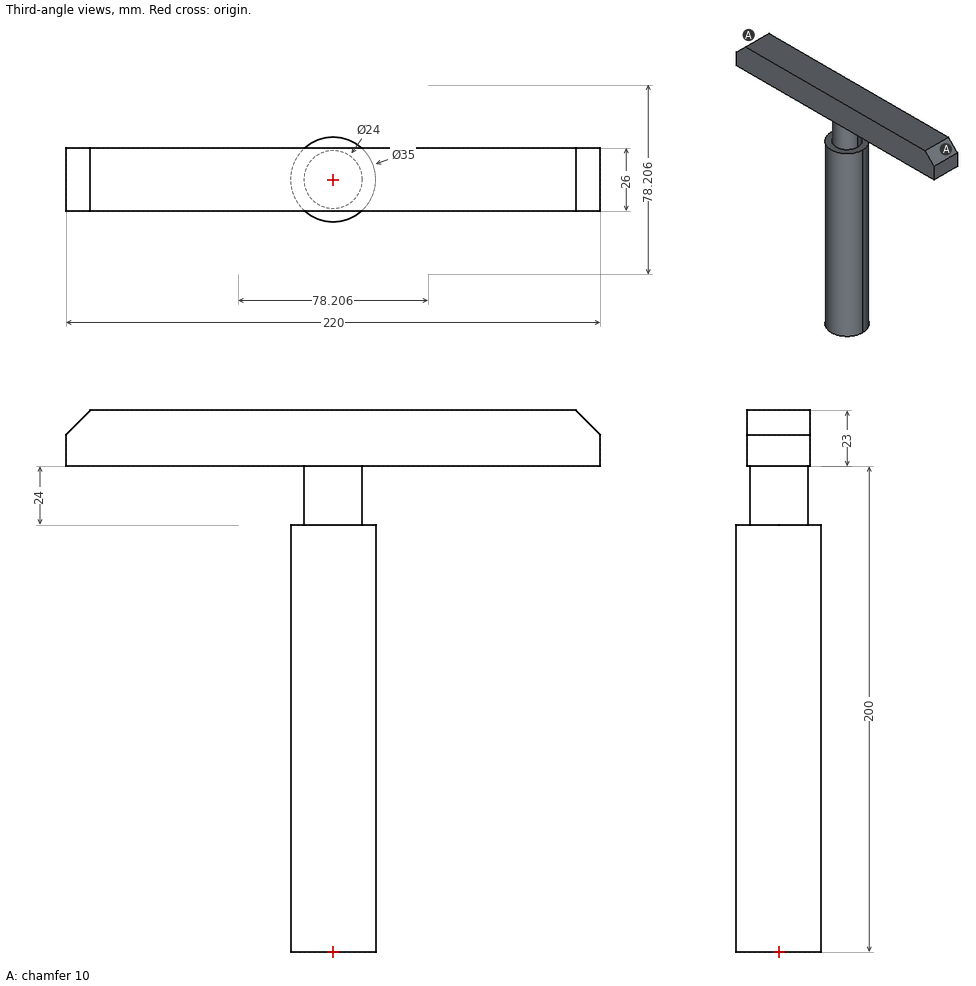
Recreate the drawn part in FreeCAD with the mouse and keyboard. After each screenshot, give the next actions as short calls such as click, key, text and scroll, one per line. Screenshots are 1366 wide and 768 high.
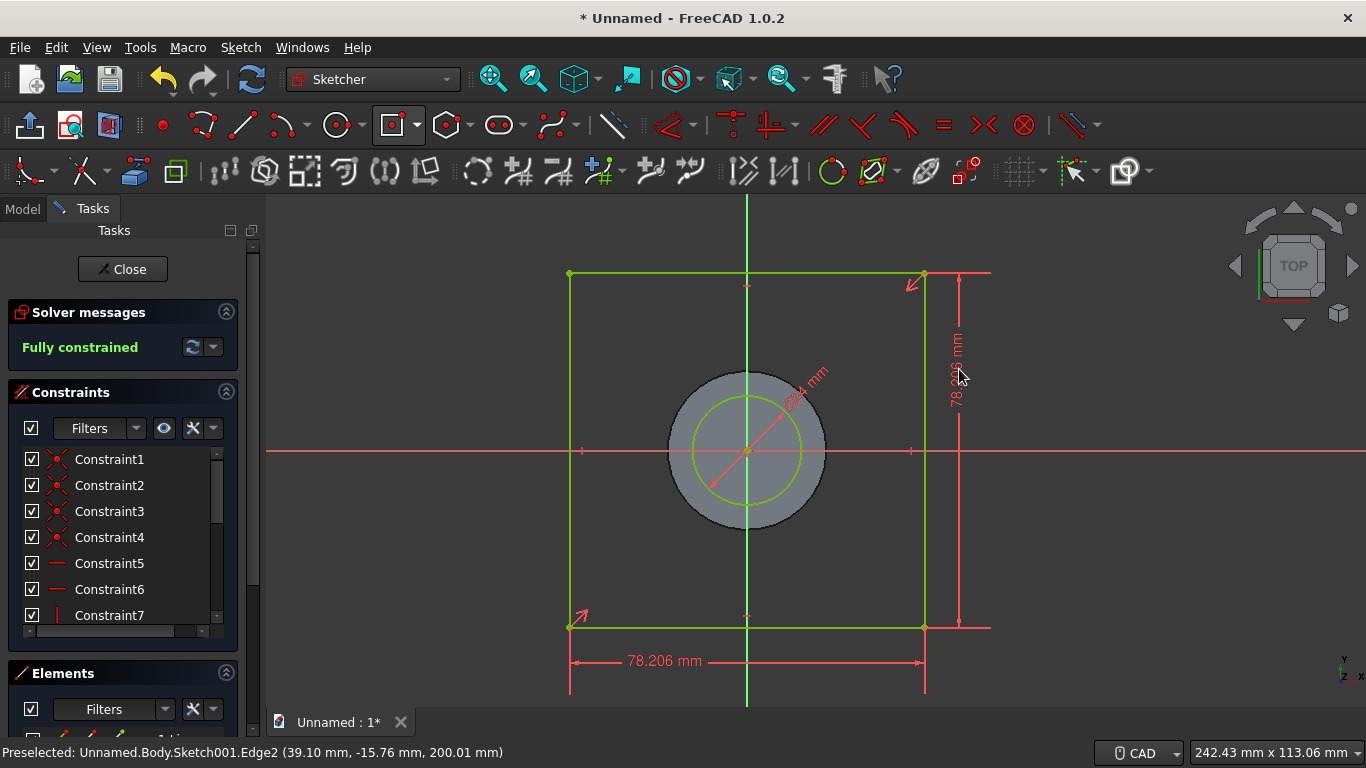
click(123, 269)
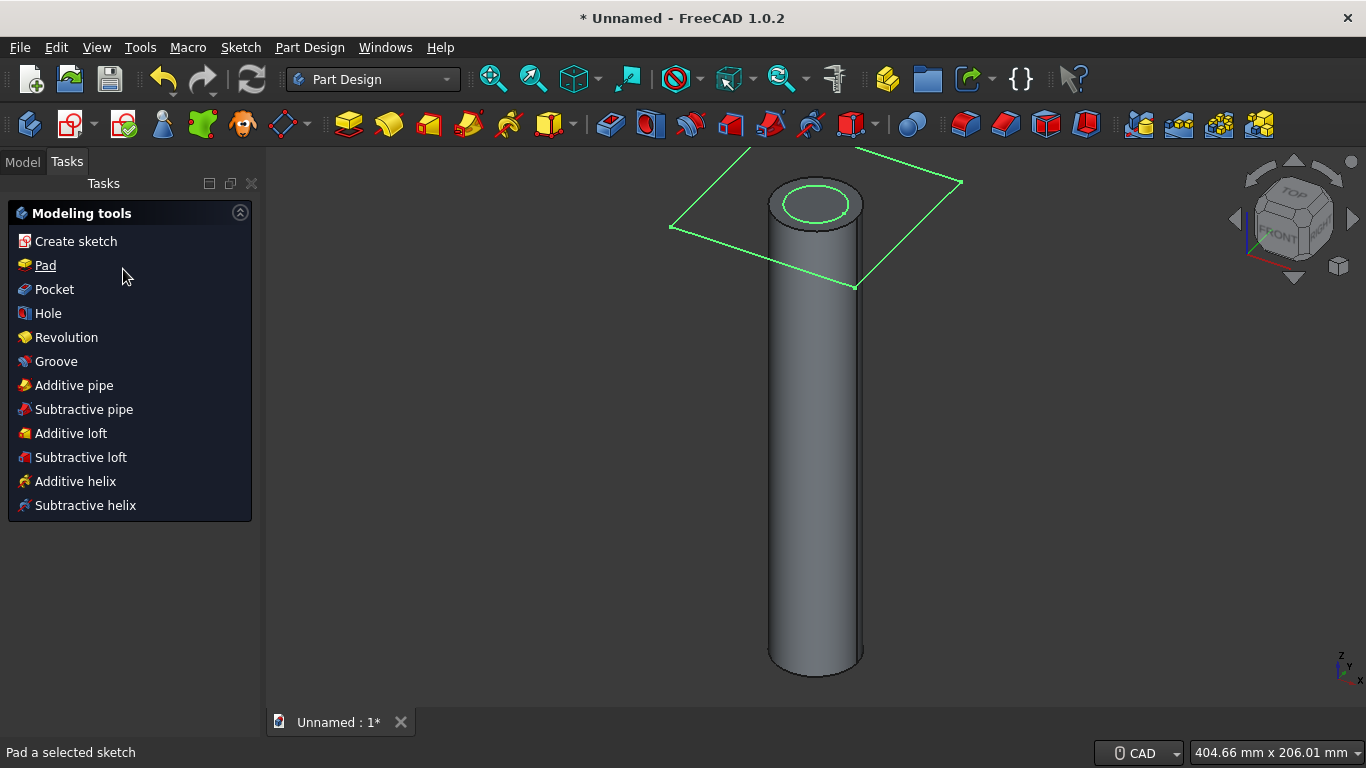
click(612, 124)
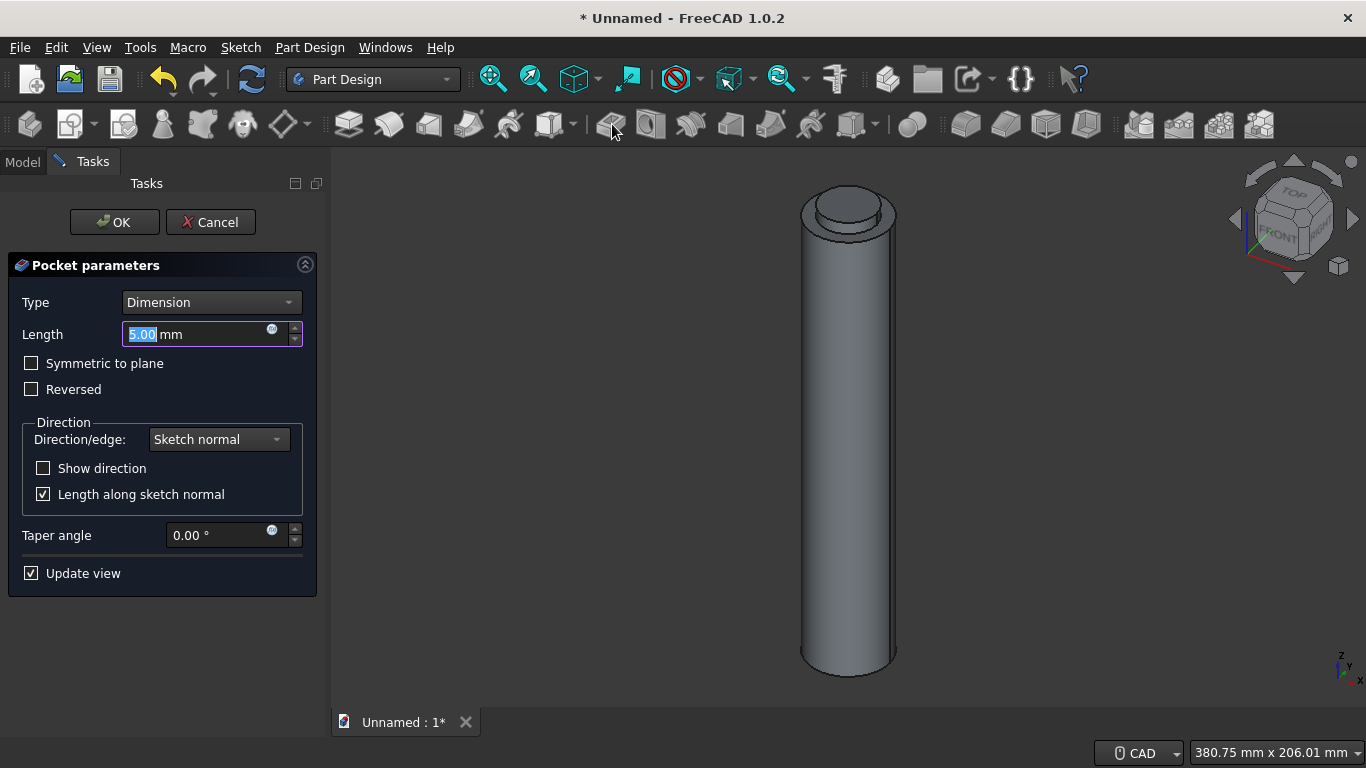
text(24)
key(Tab)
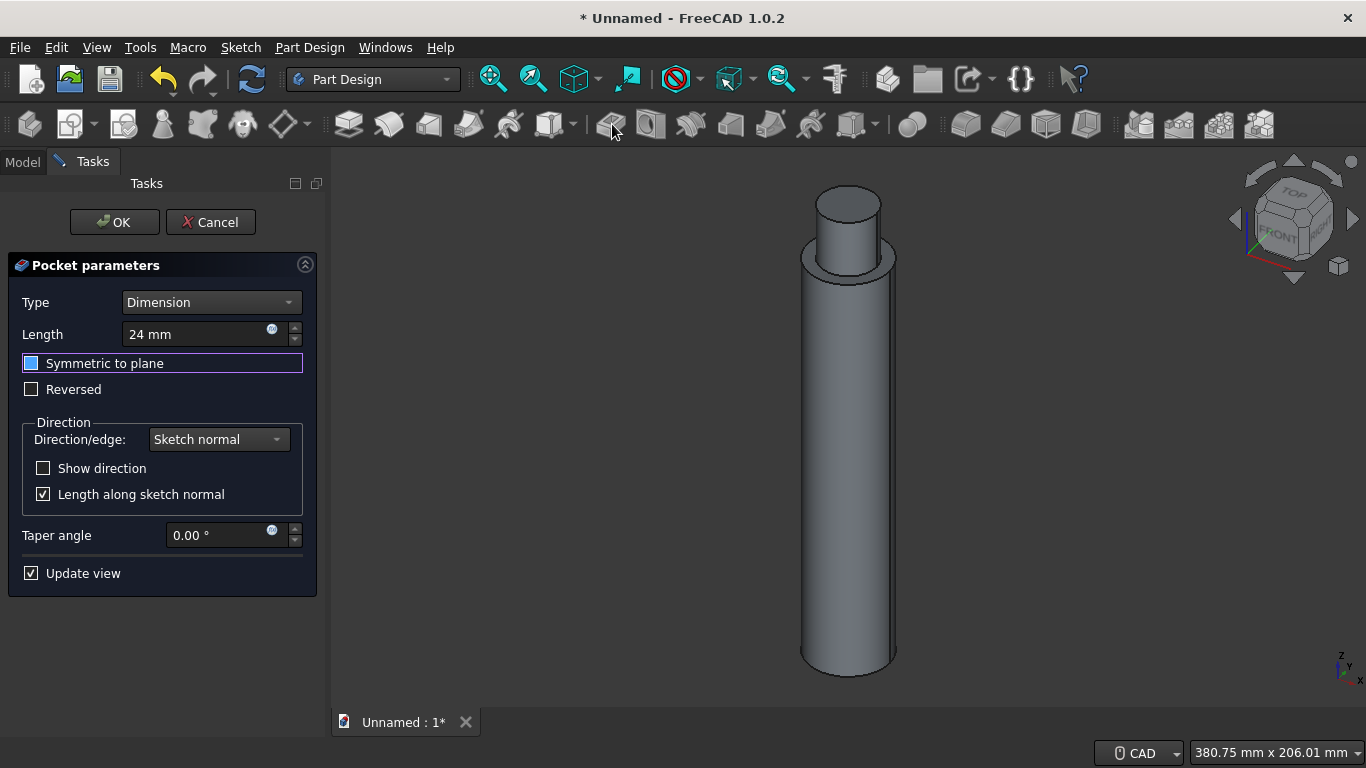
click(115, 222)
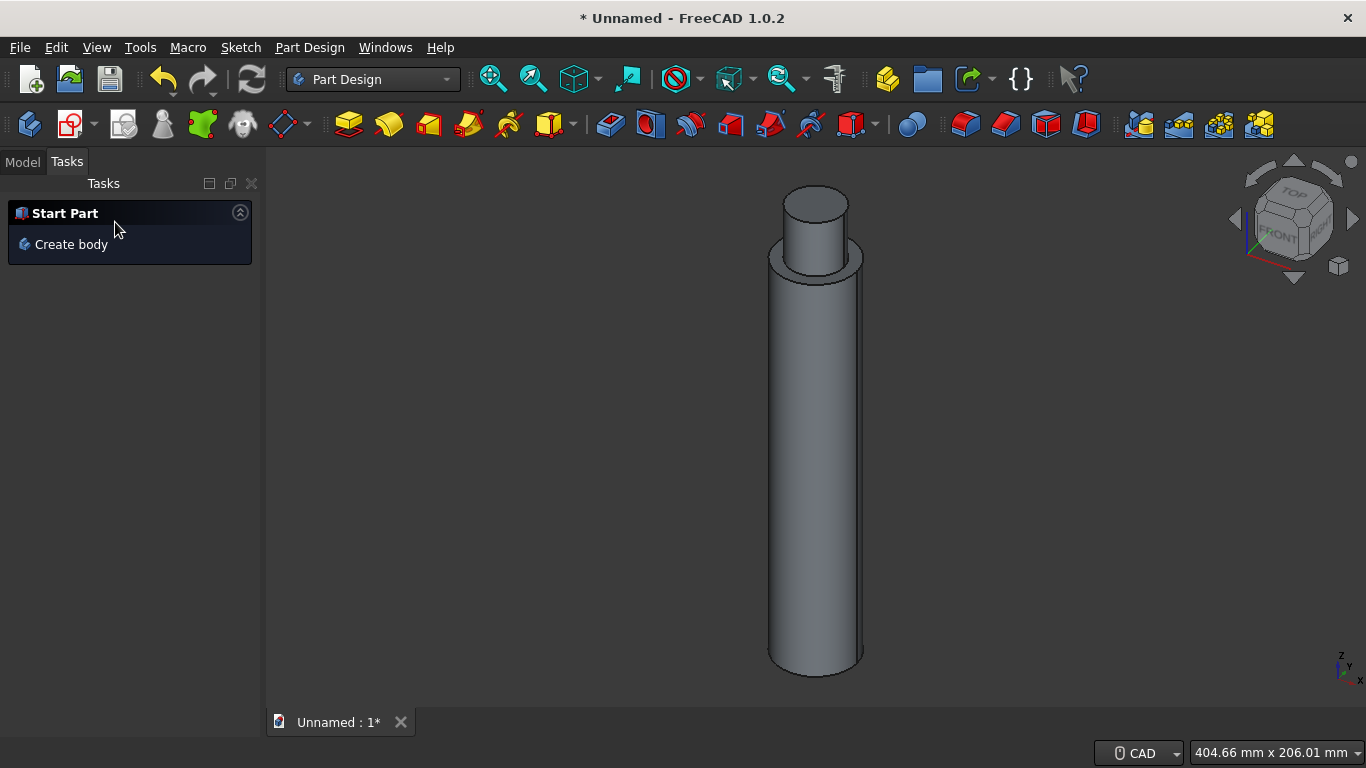
click(816, 203)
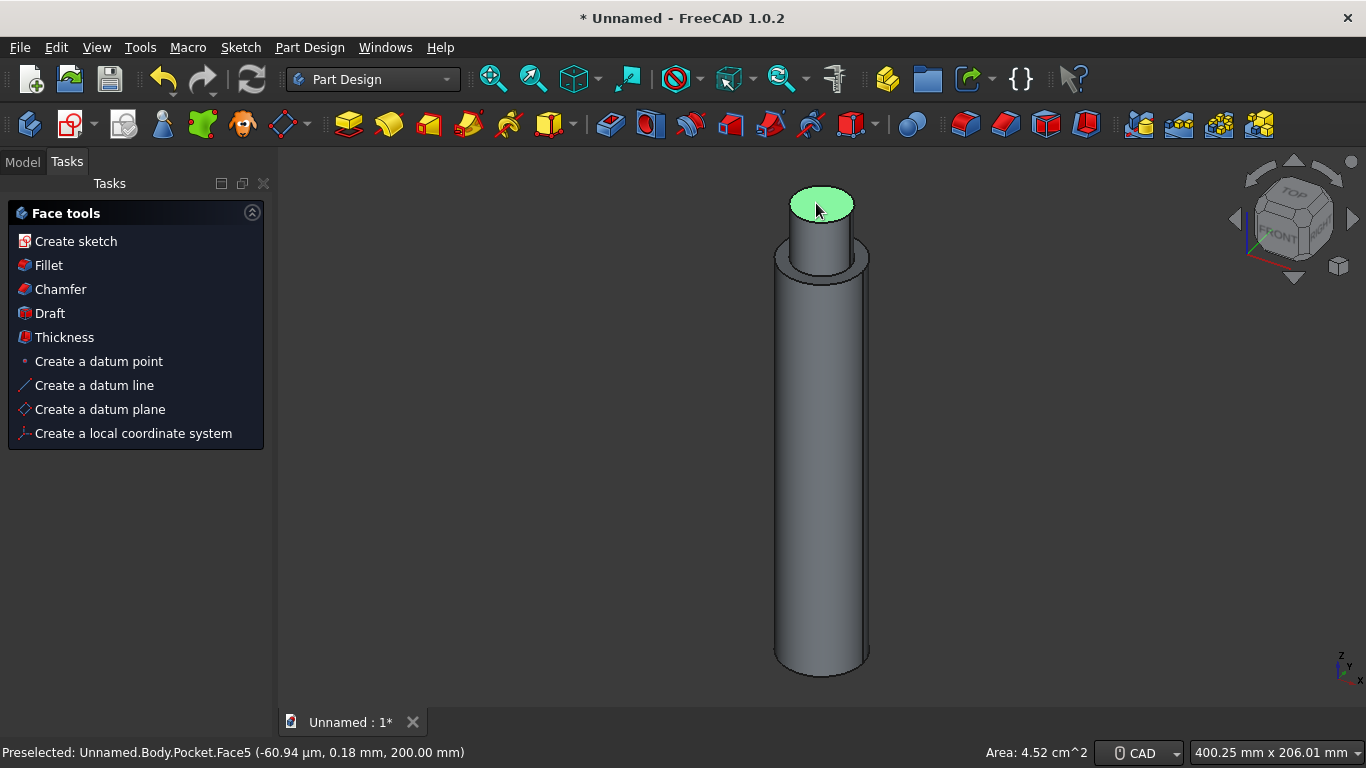
click(70, 124)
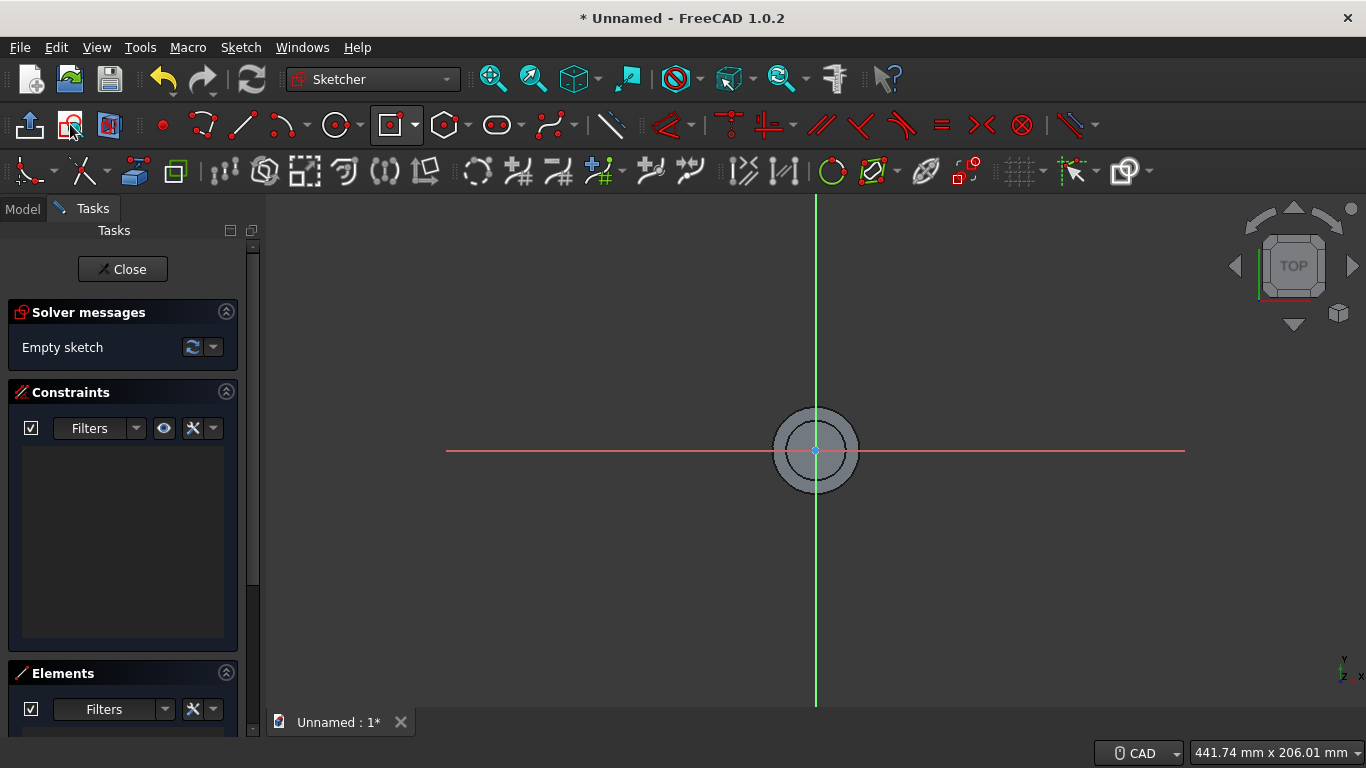
key(g)
key(v)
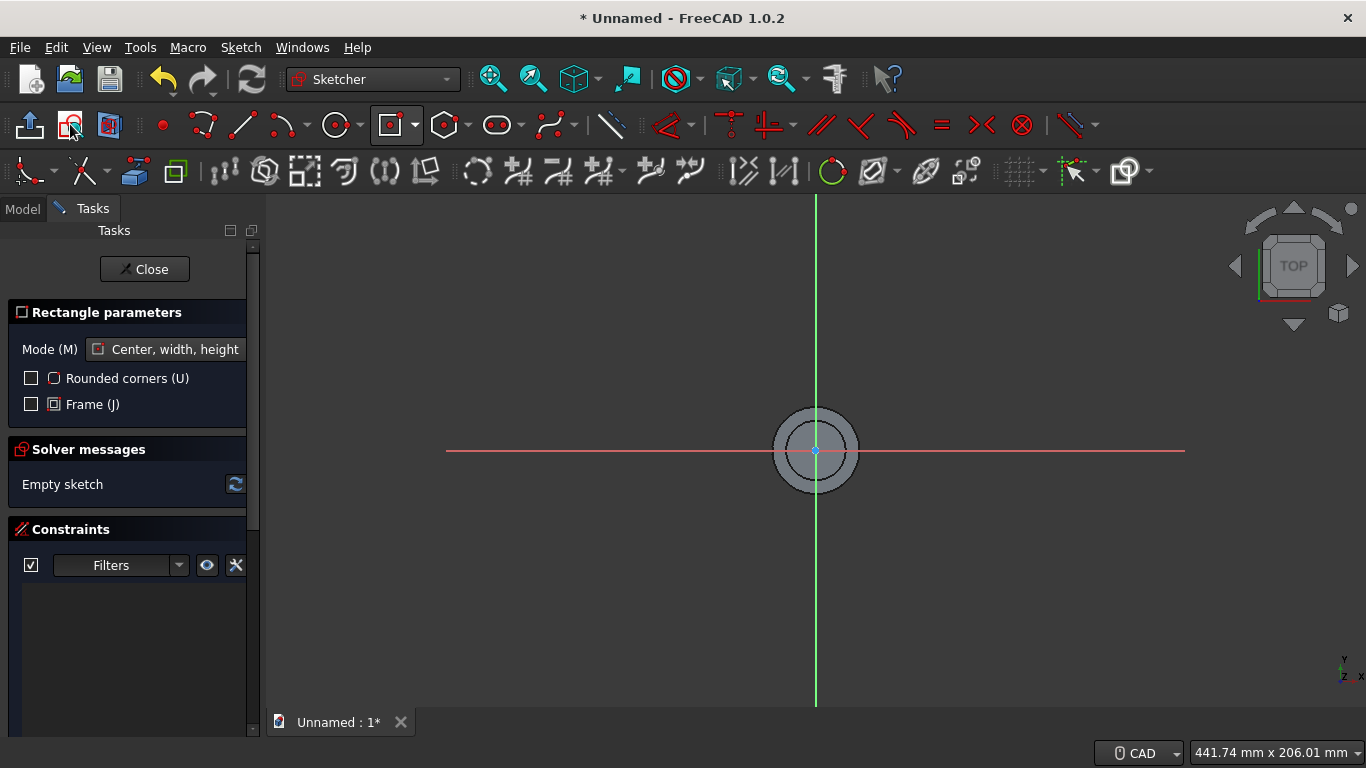
click(816, 450)
click(1090, 418)
key(Escape)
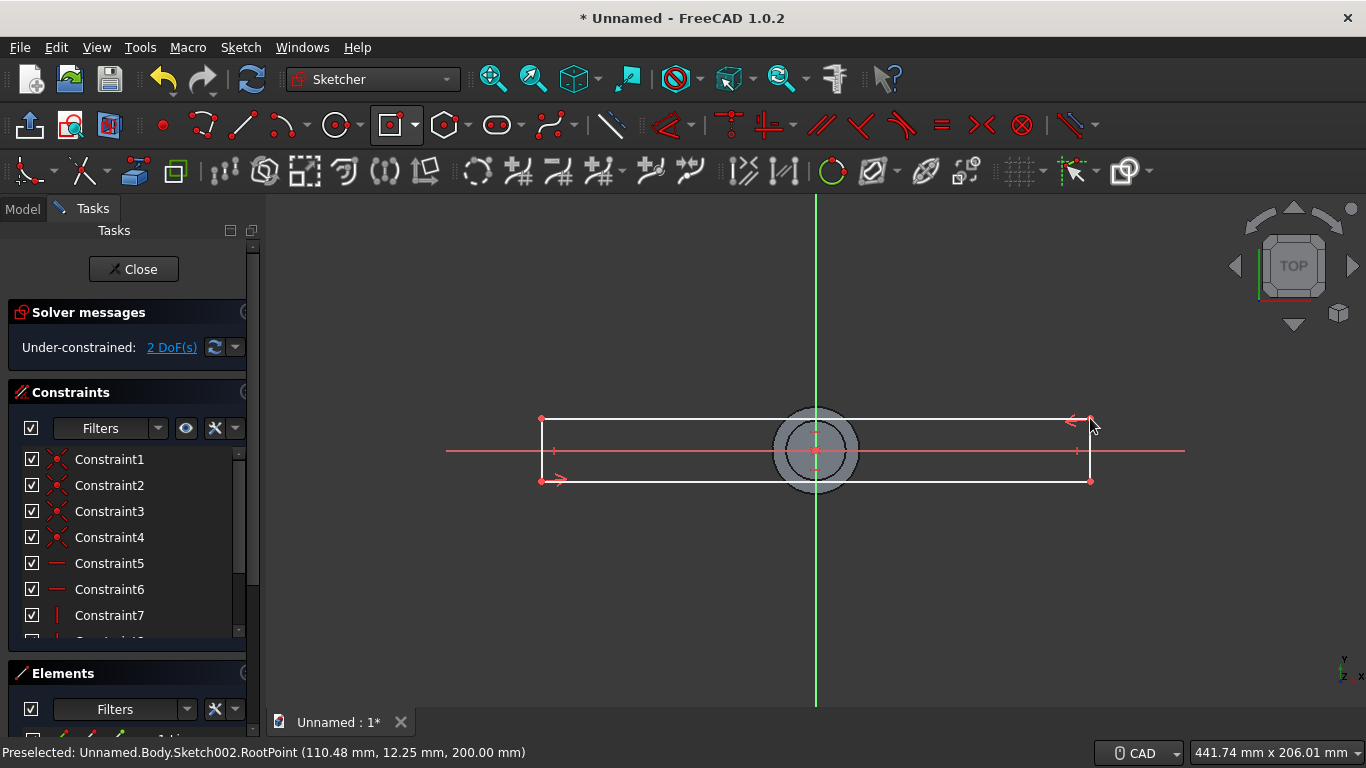
click(666, 126)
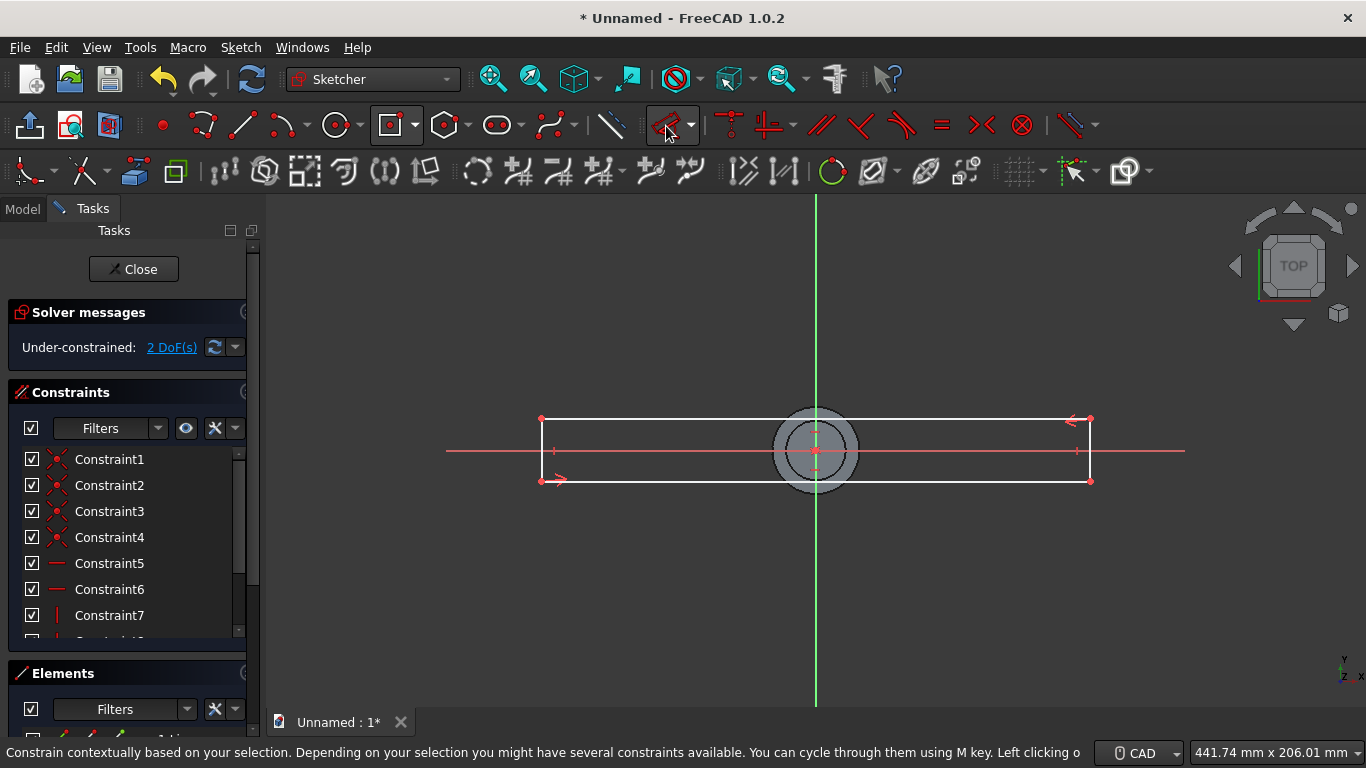
click(1090, 463)
click(1124, 436)